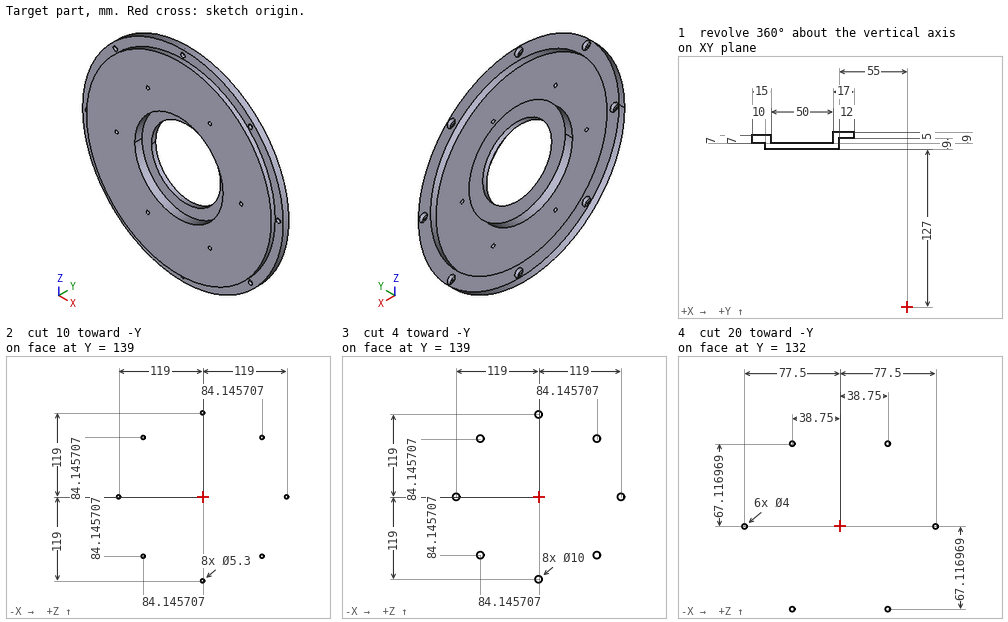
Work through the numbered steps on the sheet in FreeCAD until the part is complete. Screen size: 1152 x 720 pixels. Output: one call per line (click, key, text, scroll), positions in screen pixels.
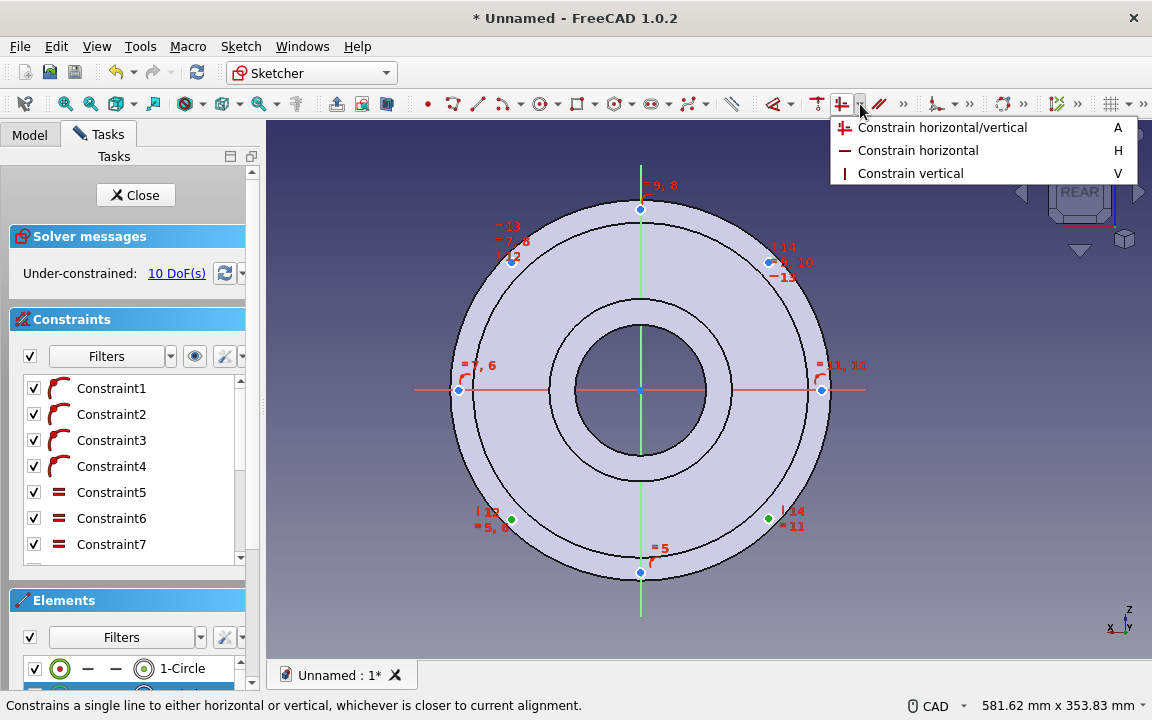
click(984, 150)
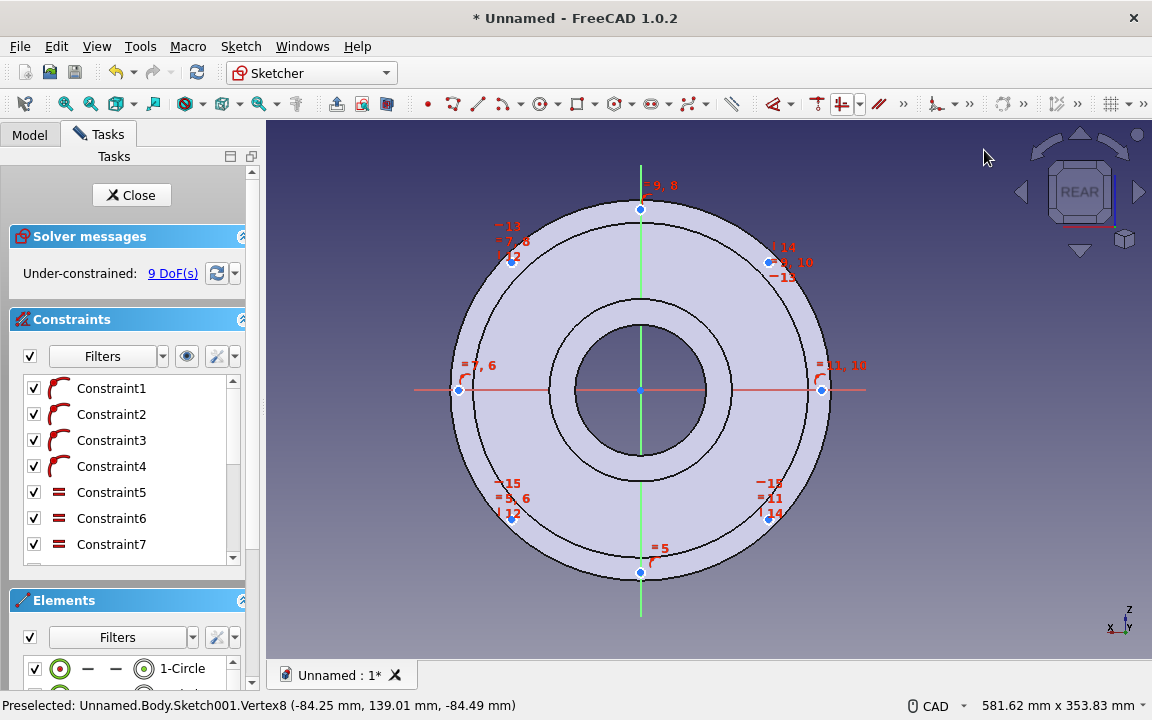
click(772, 104)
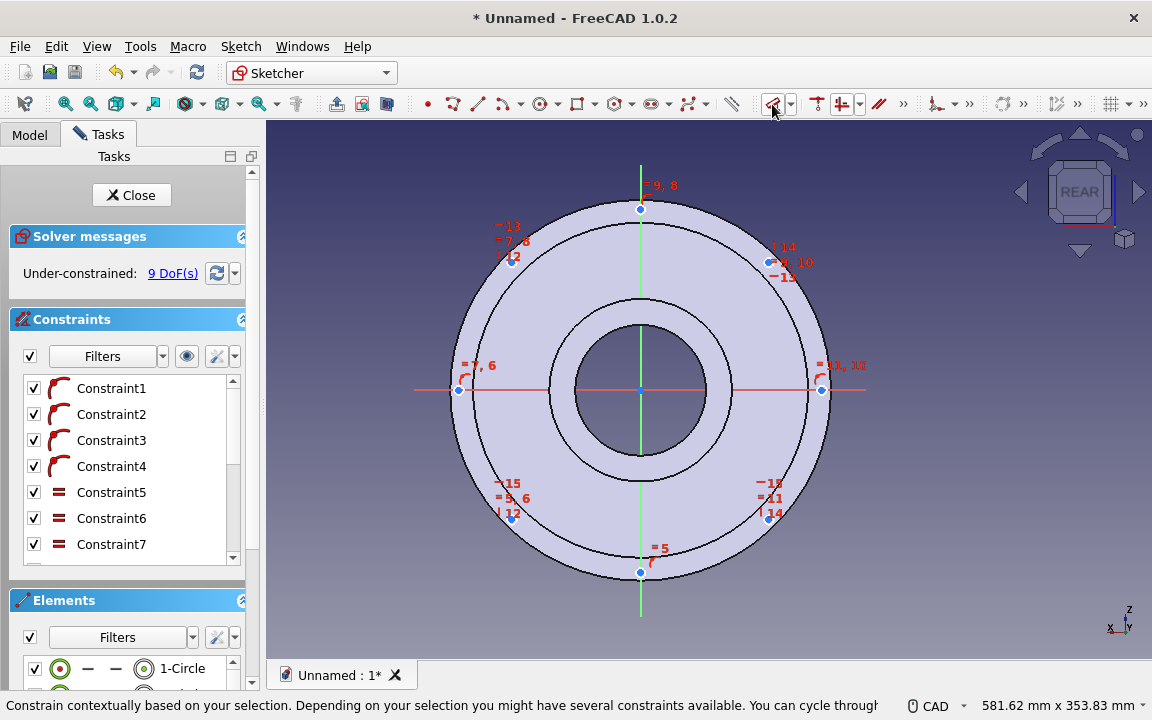
scroll(641, 568, up, 8)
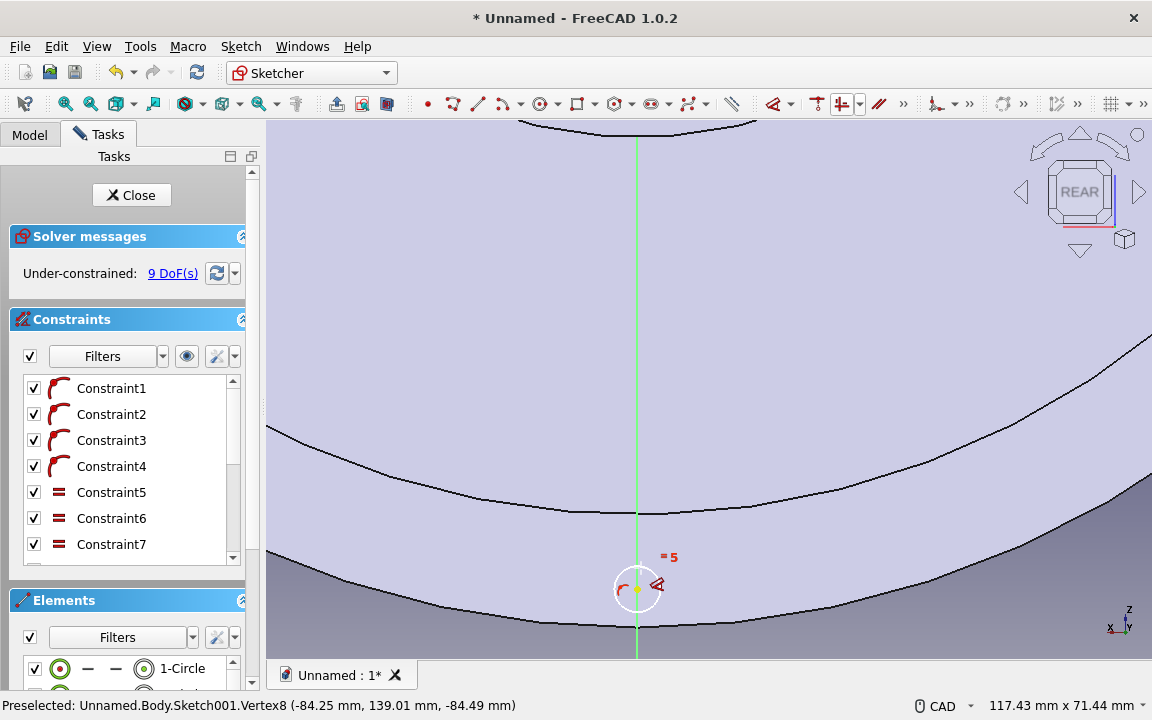
click(638, 566)
click(665, 541)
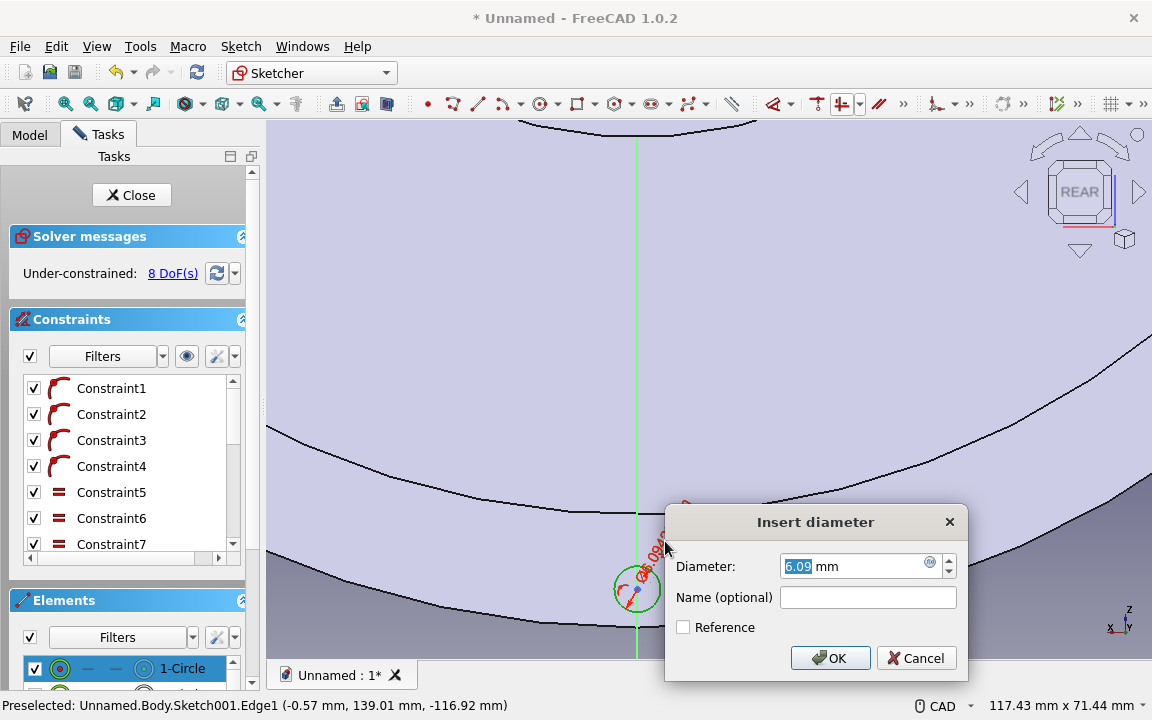
text(5.3)
key(Return)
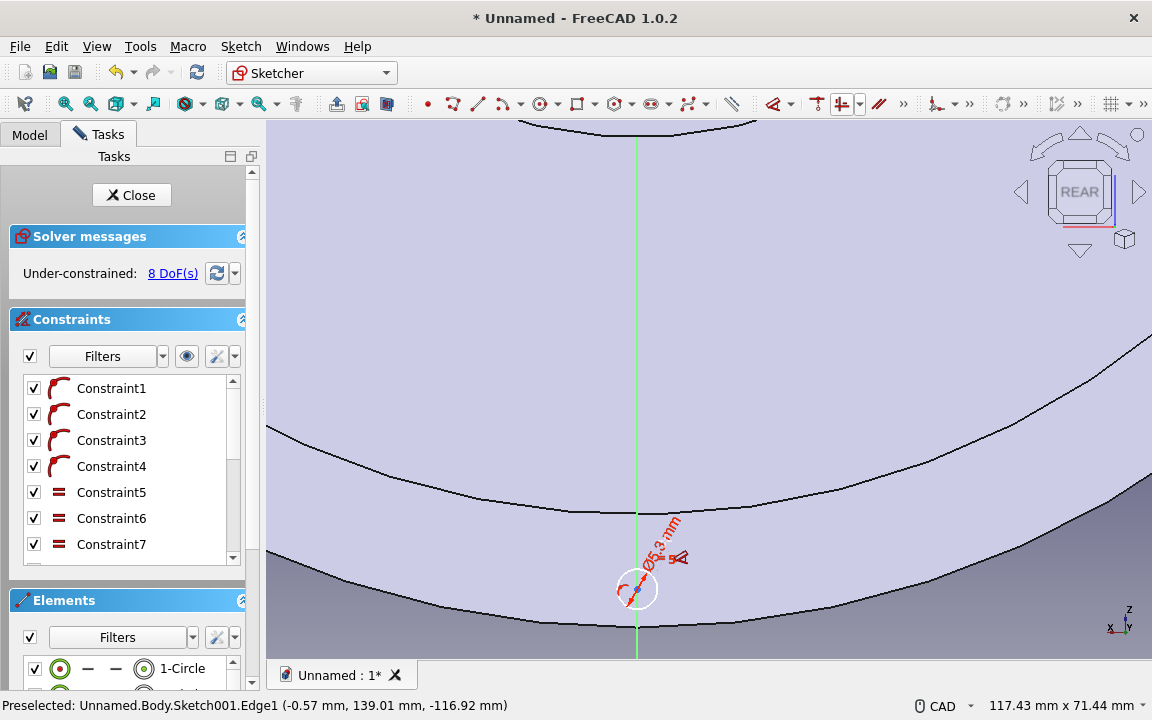
scroll(641, 568, down, 8)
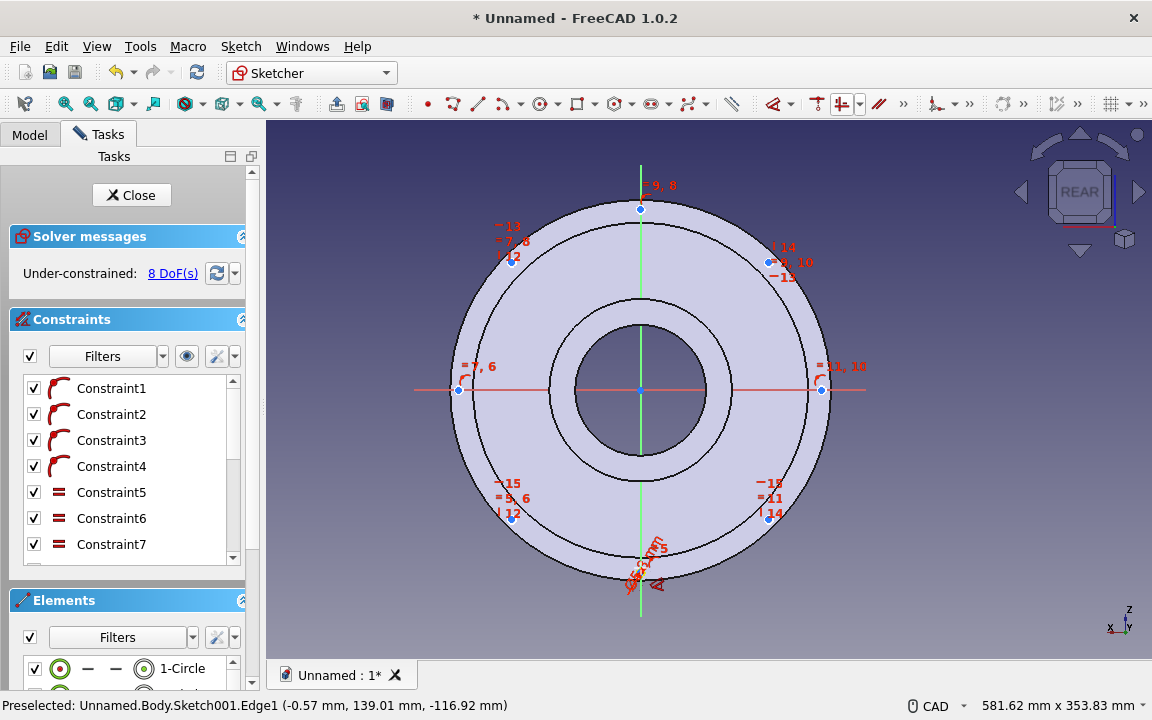
click(641, 573)
click(675, 482)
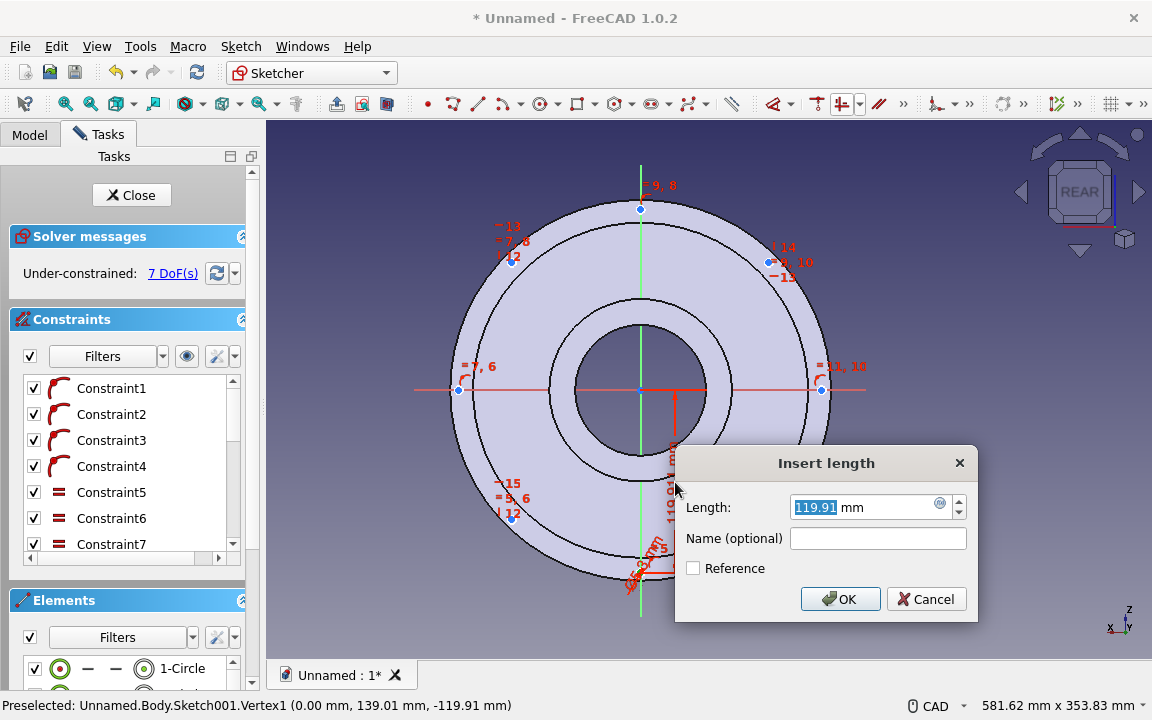
text(119)
key(Return)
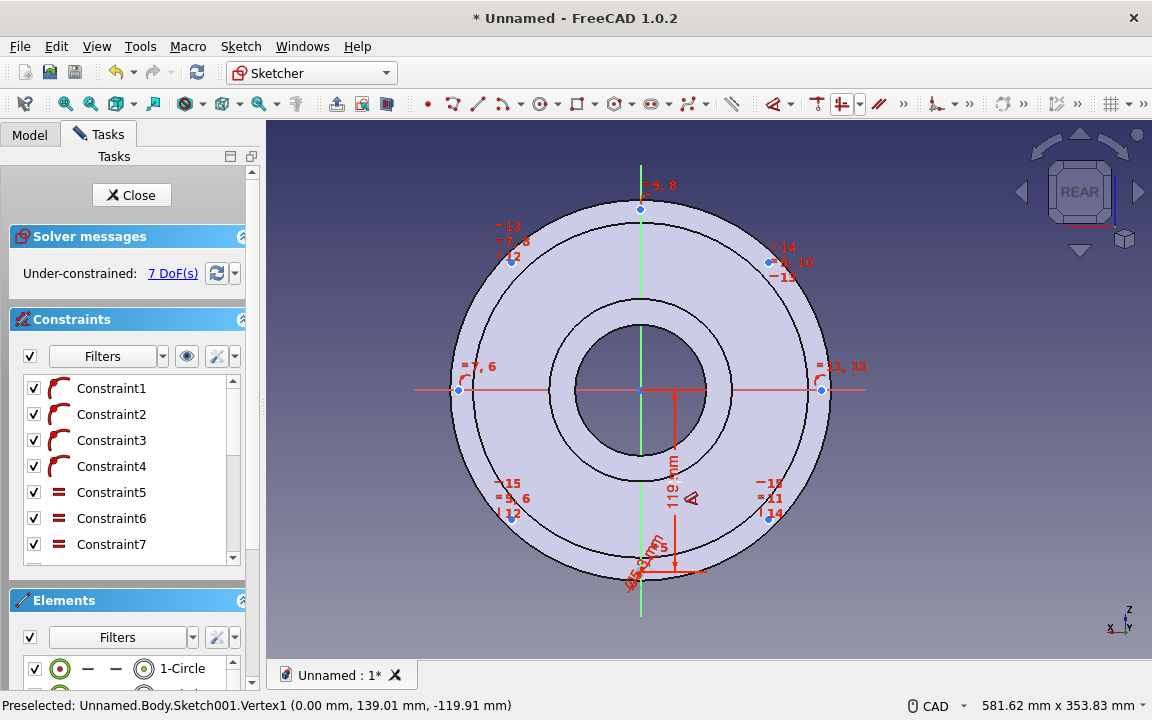
click(459, 390)
click(550, 424)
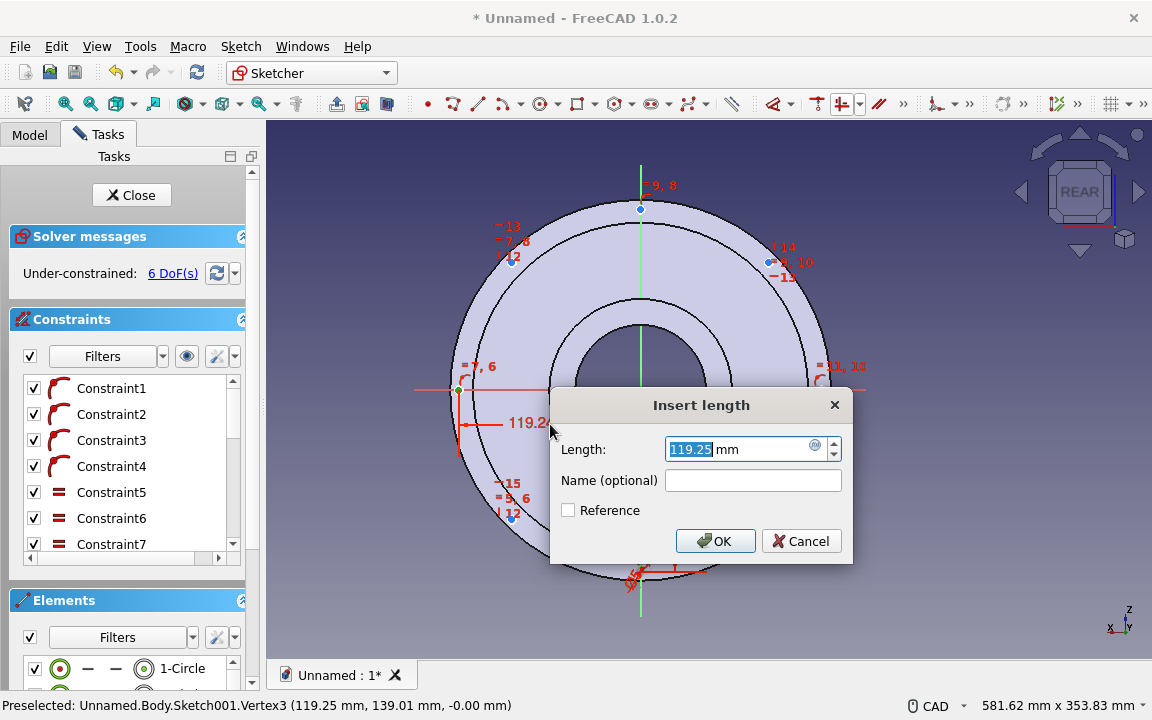
text(119)
key(Return)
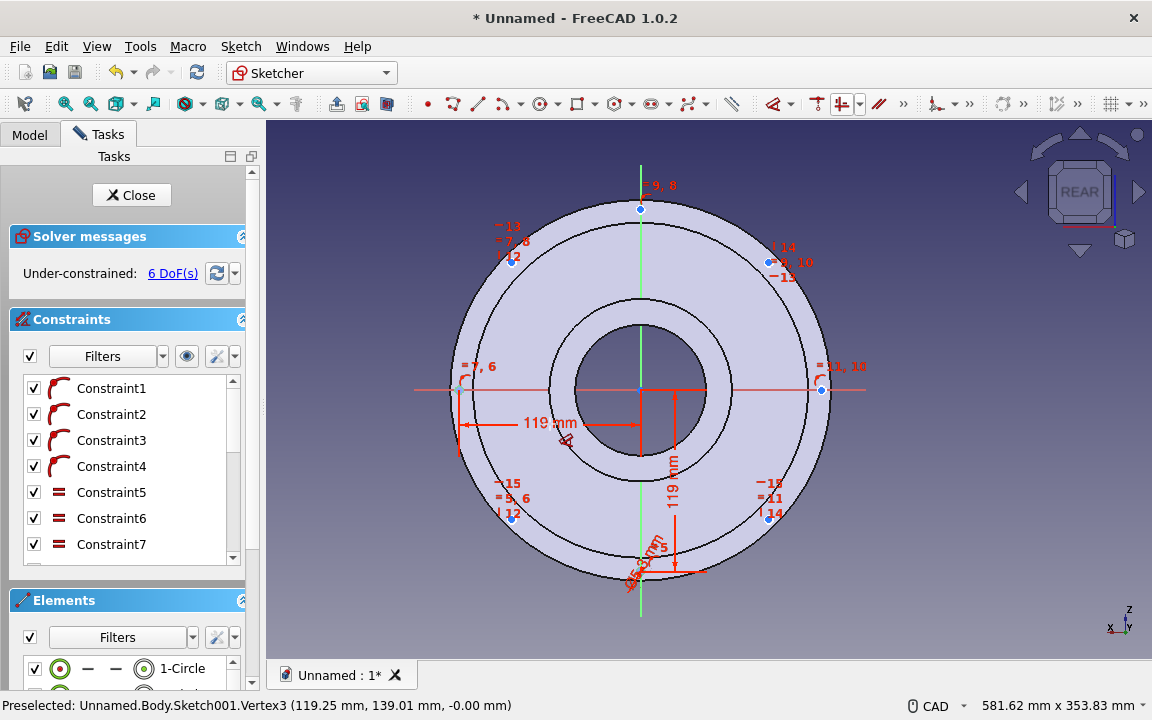
click(641, 210)
click(675, 300)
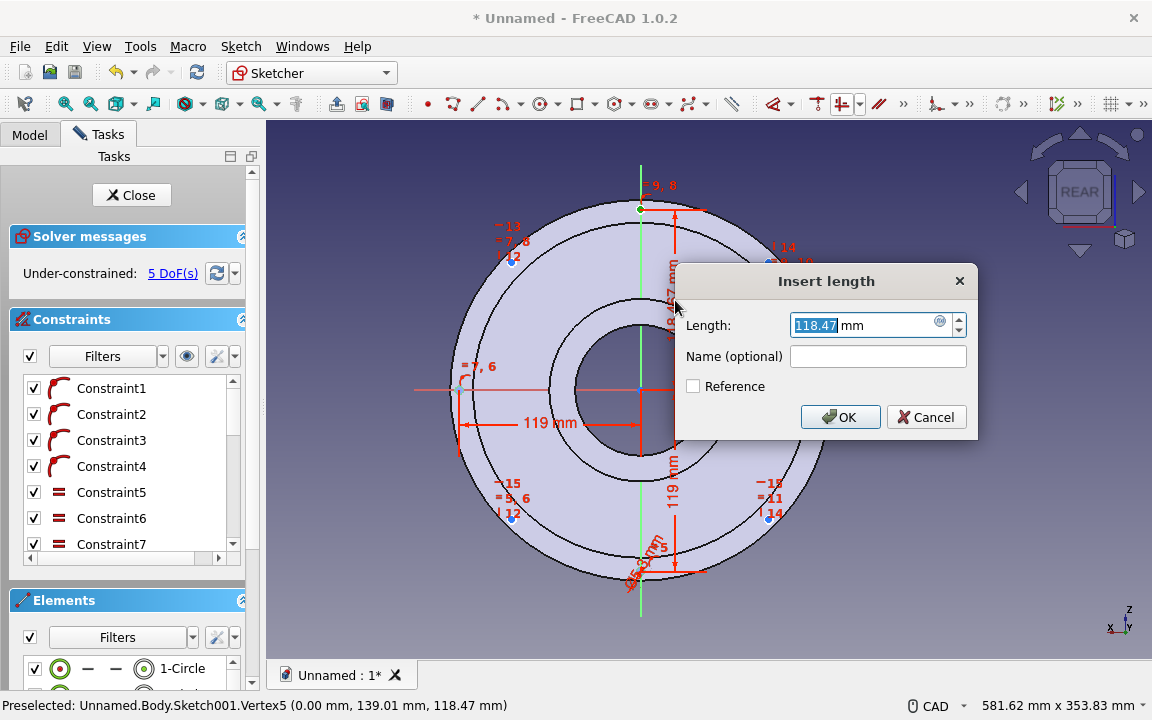
text(119)
key(Return)